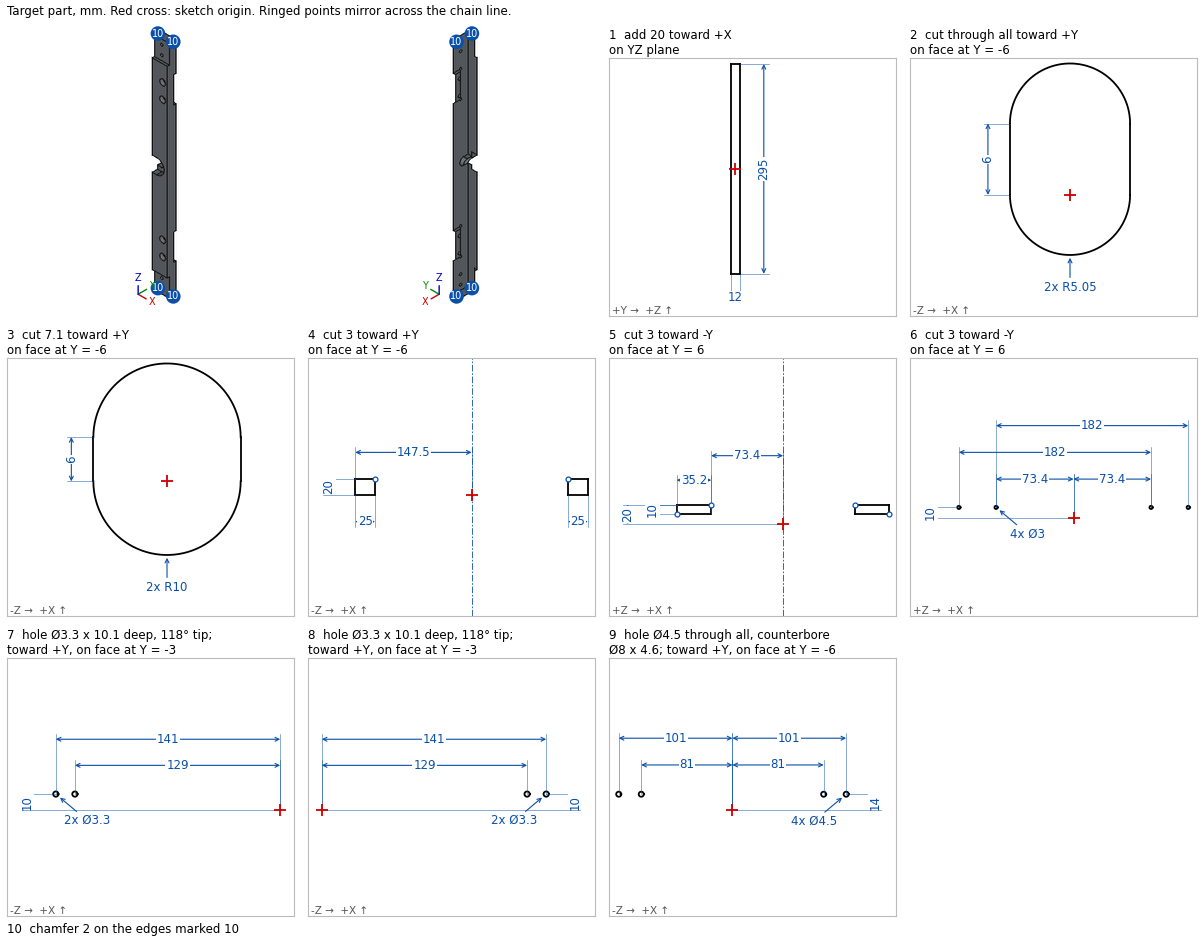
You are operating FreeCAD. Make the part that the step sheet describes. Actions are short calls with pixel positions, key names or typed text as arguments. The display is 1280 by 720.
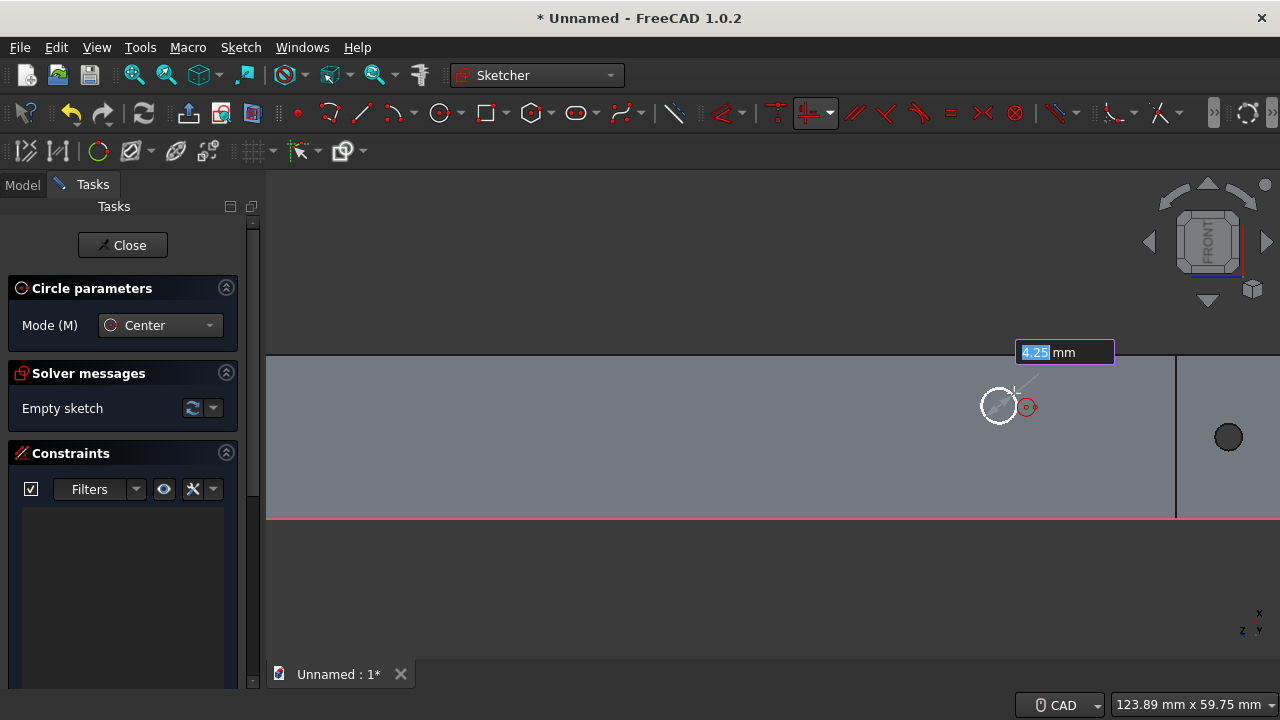
click(1013, 391)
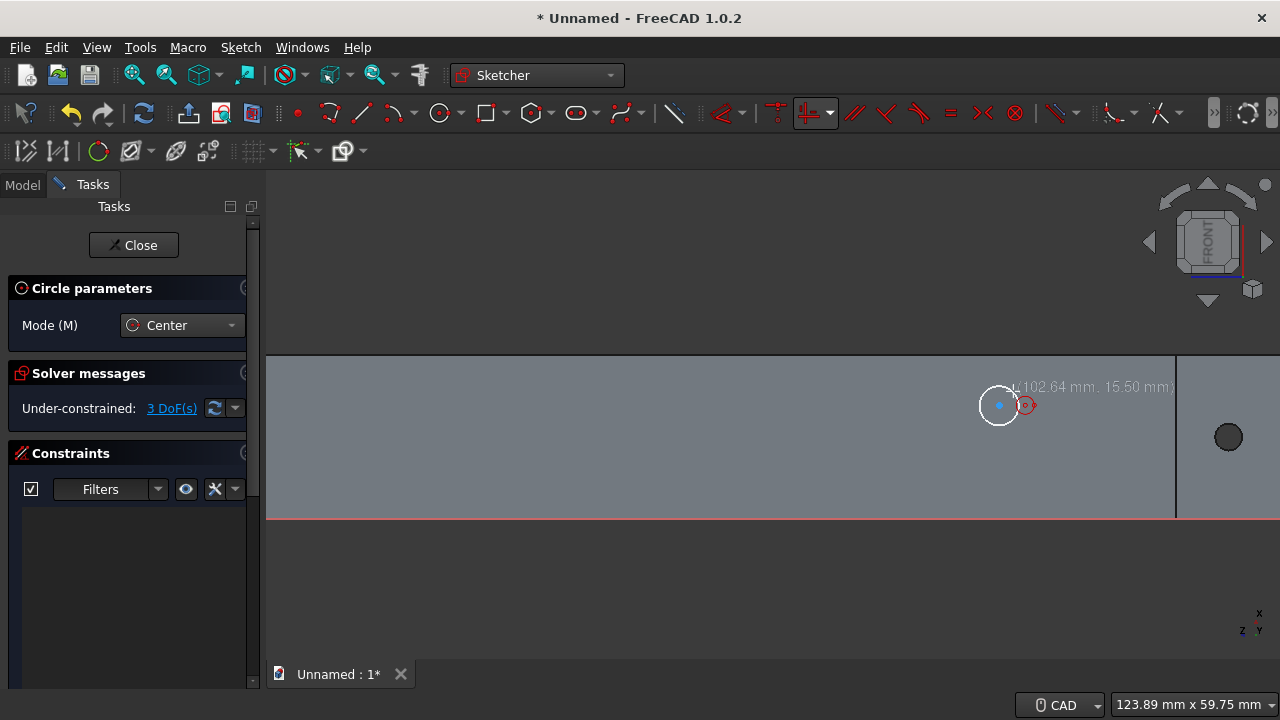
scroll(836, 404, up, 2)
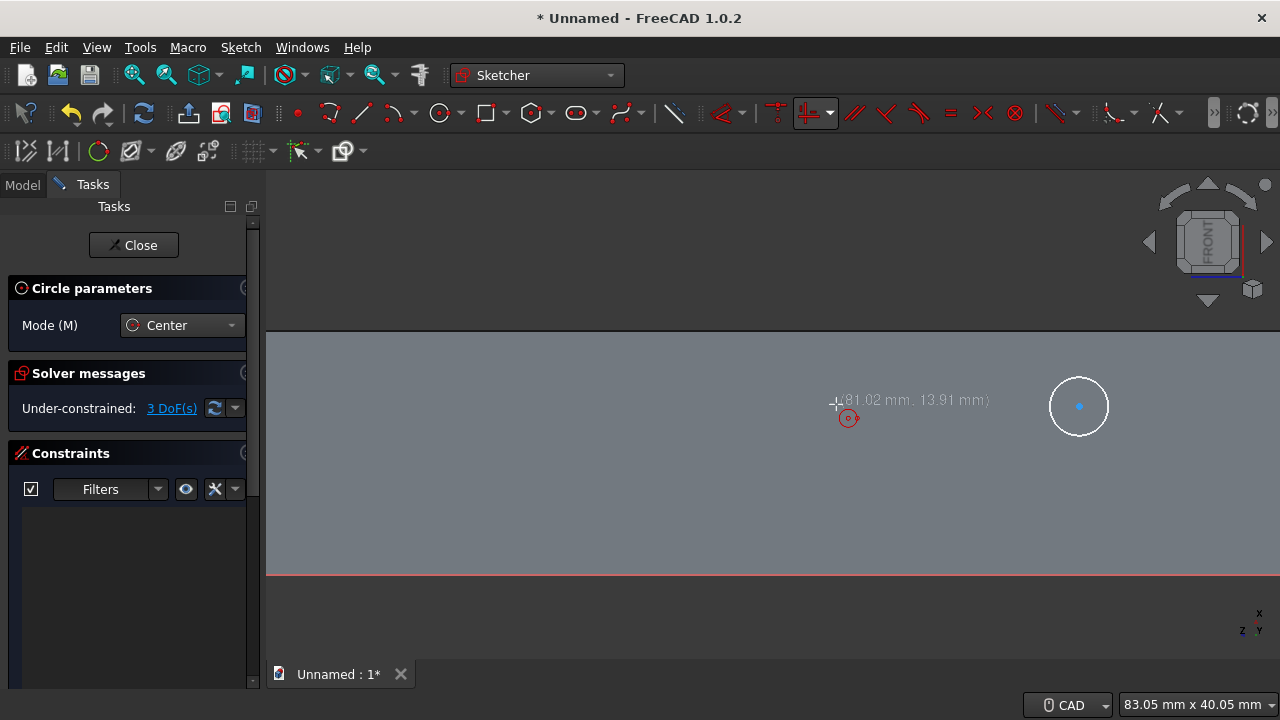
scroll(985, 394, down, 7)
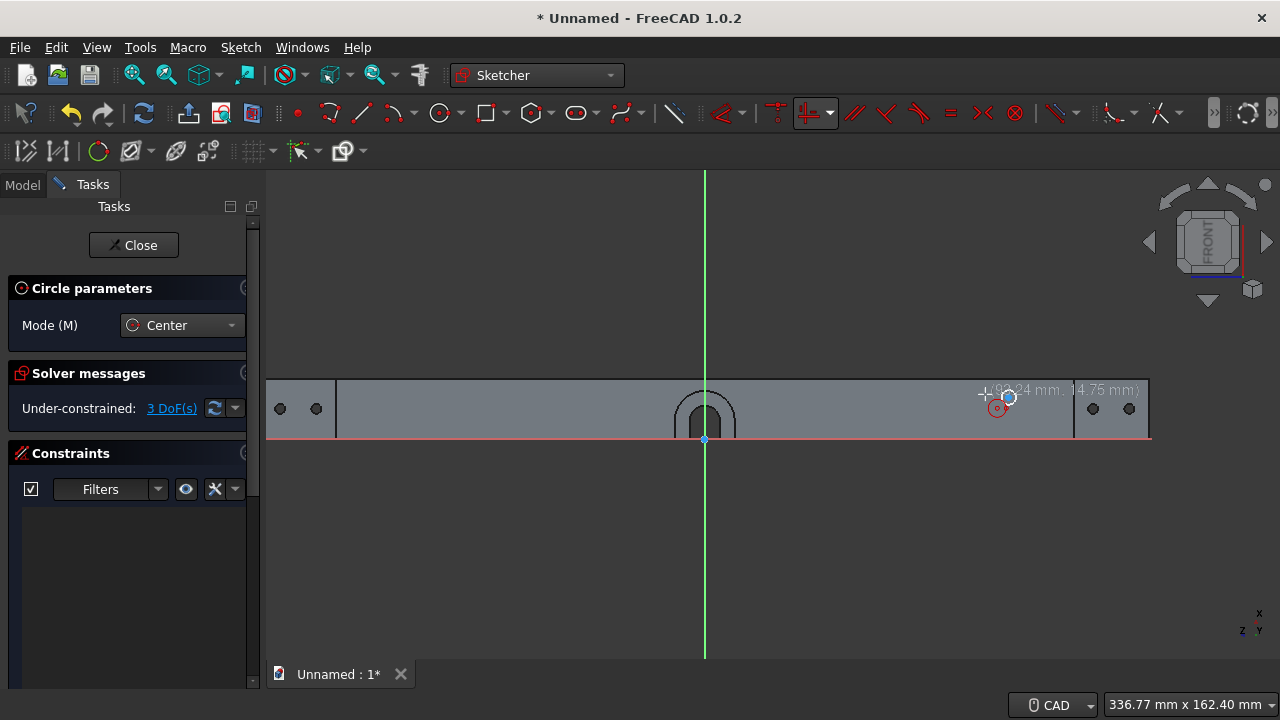
click(949, 397)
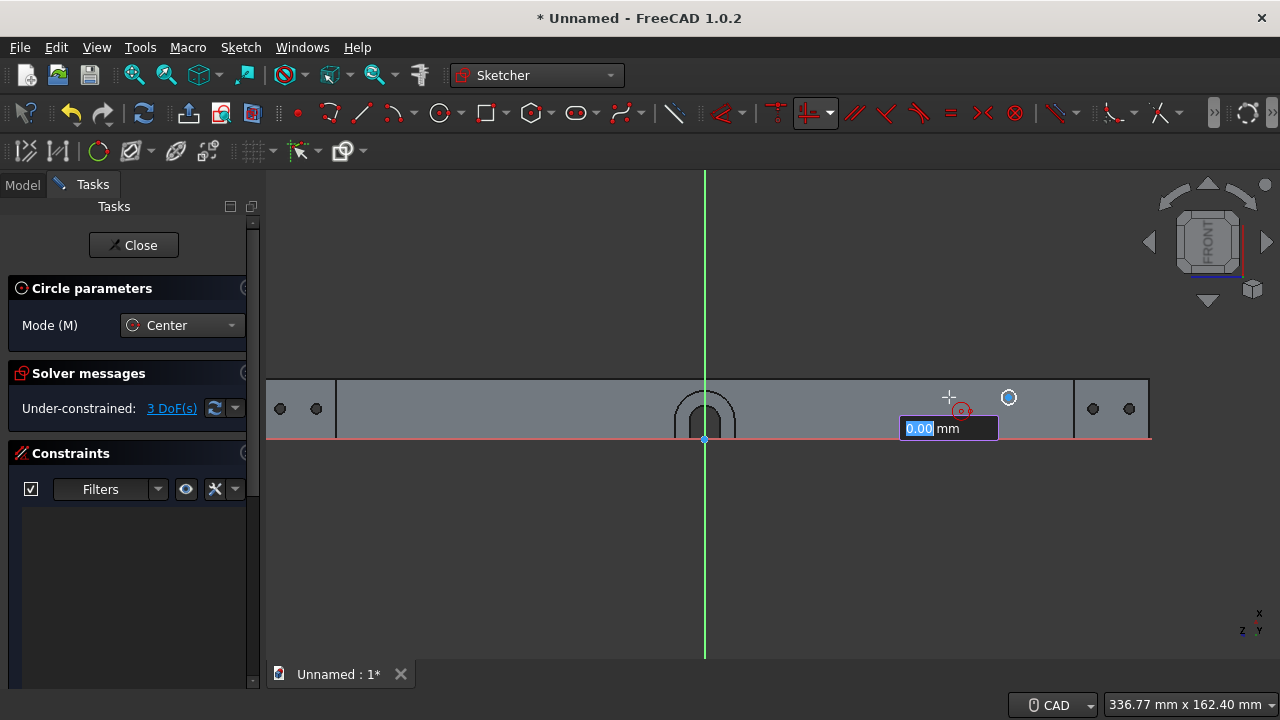
scroll(953, 392, up, 5)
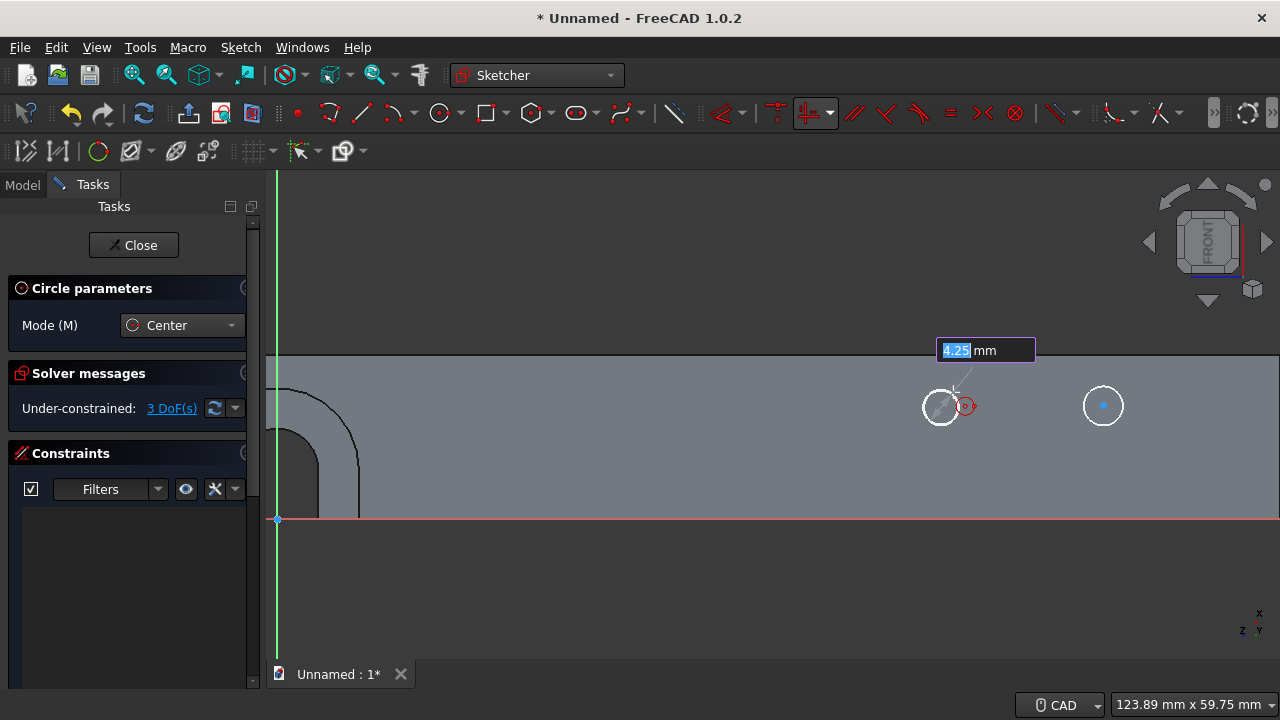
click(953, 391)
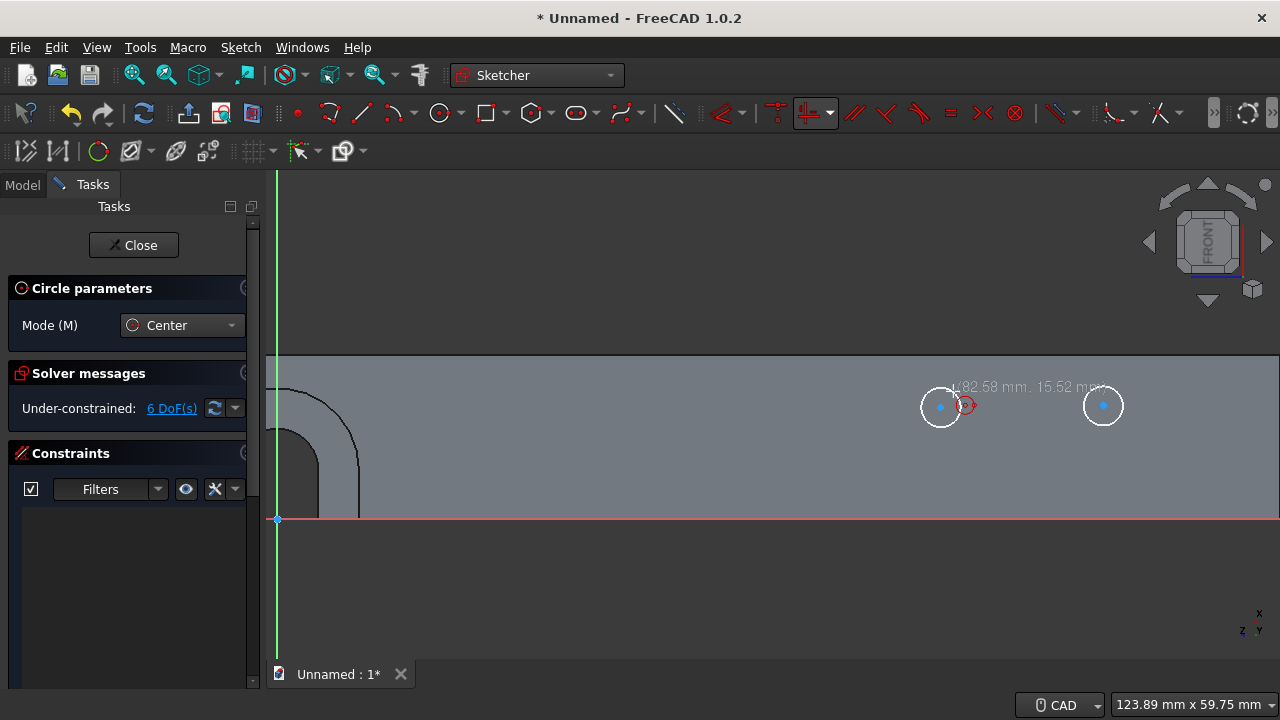
scroll(953, 392, down, 5)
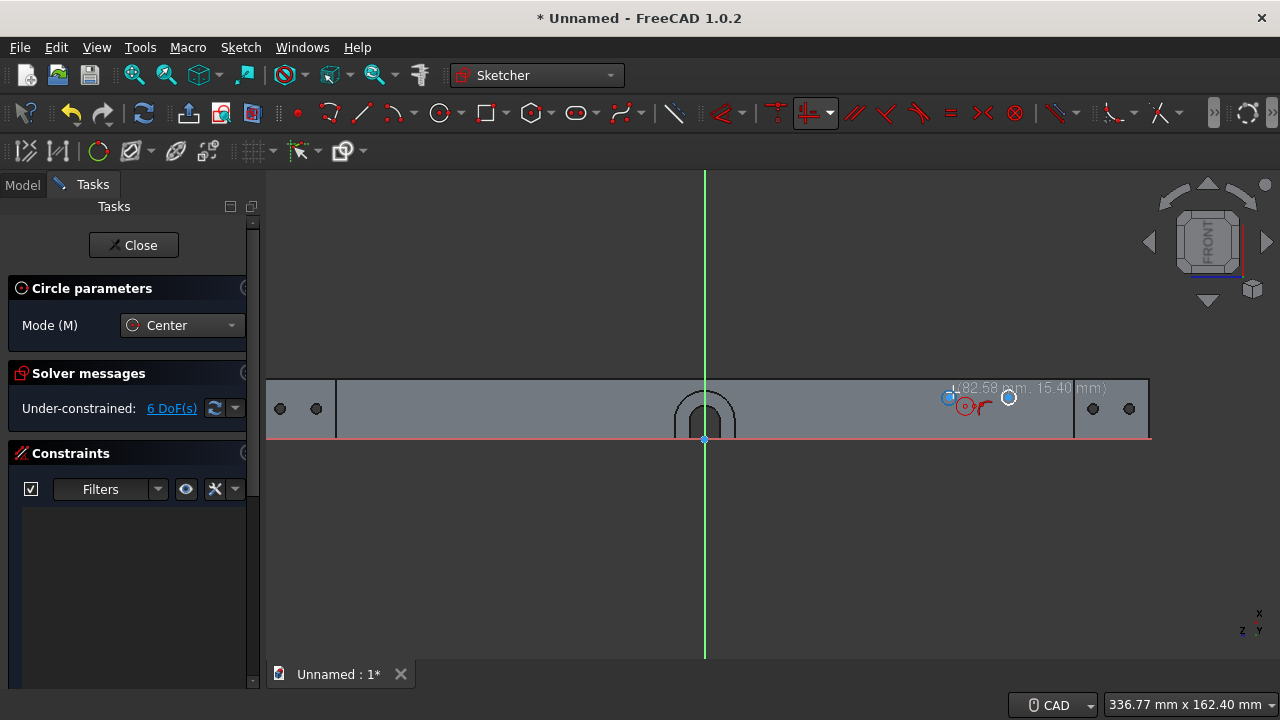
scroll(461, 397, up, 7)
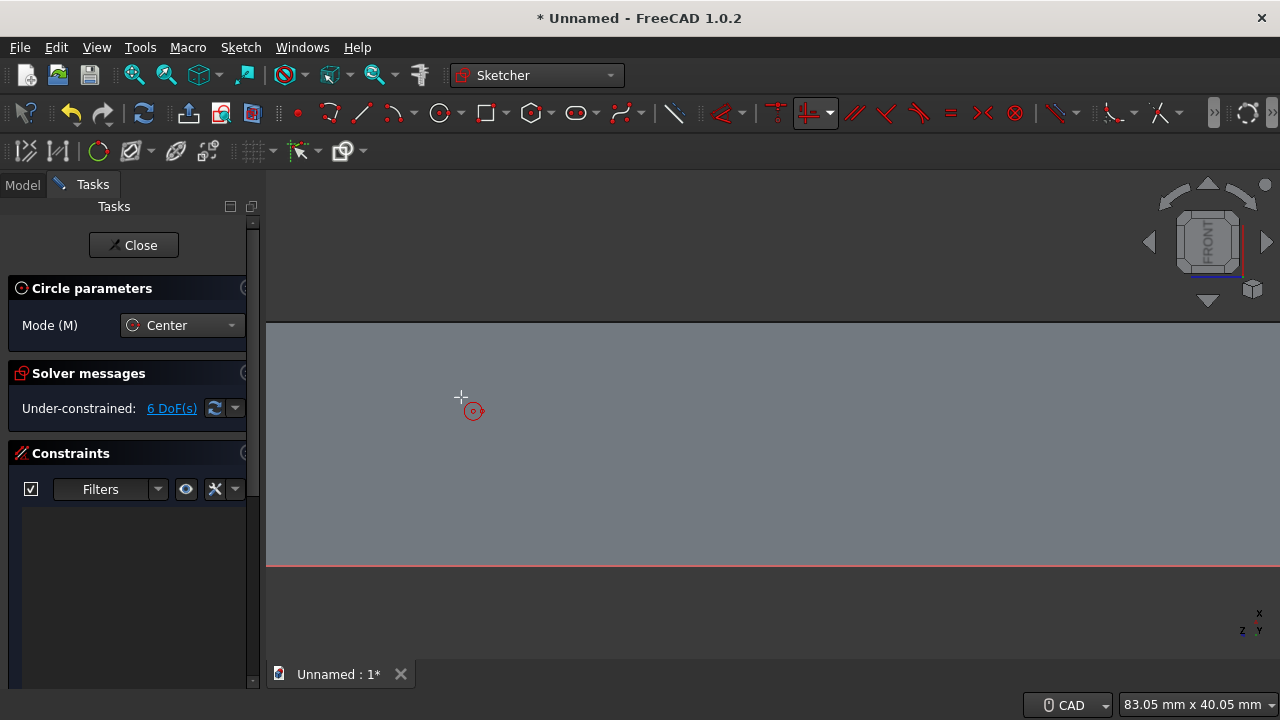
scroll(461, 397, down, 7)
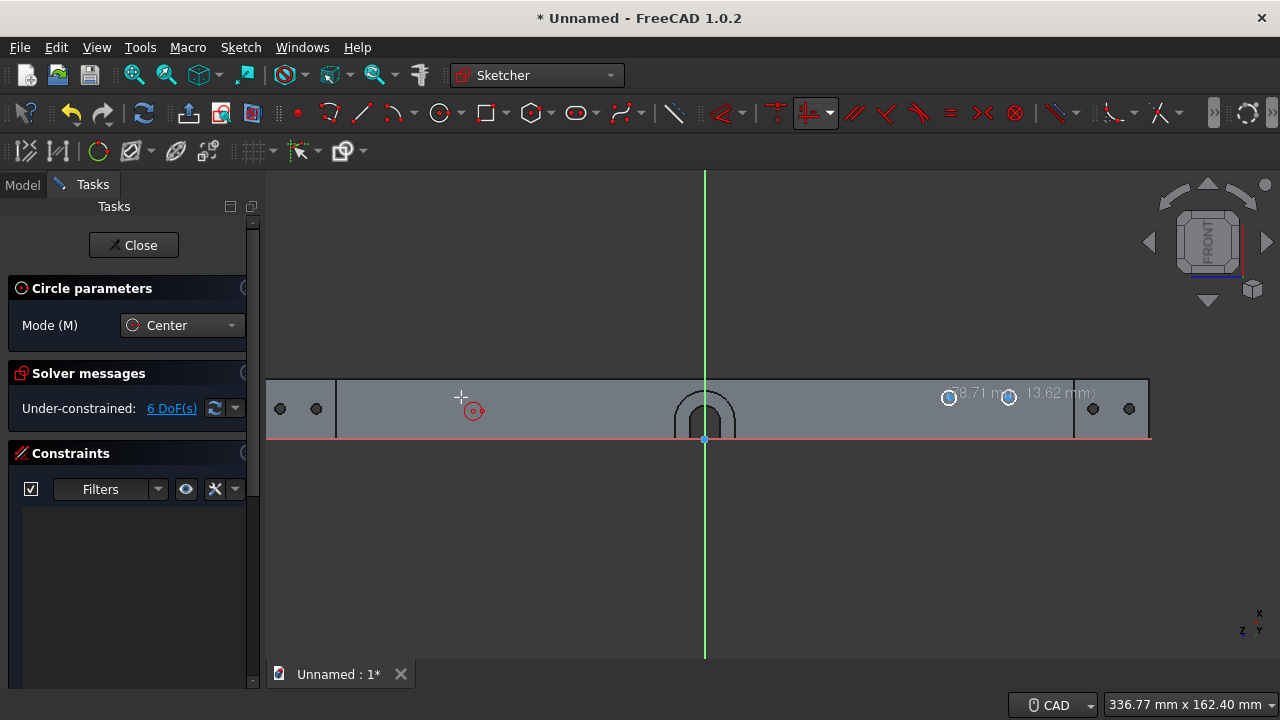
click(461, 397)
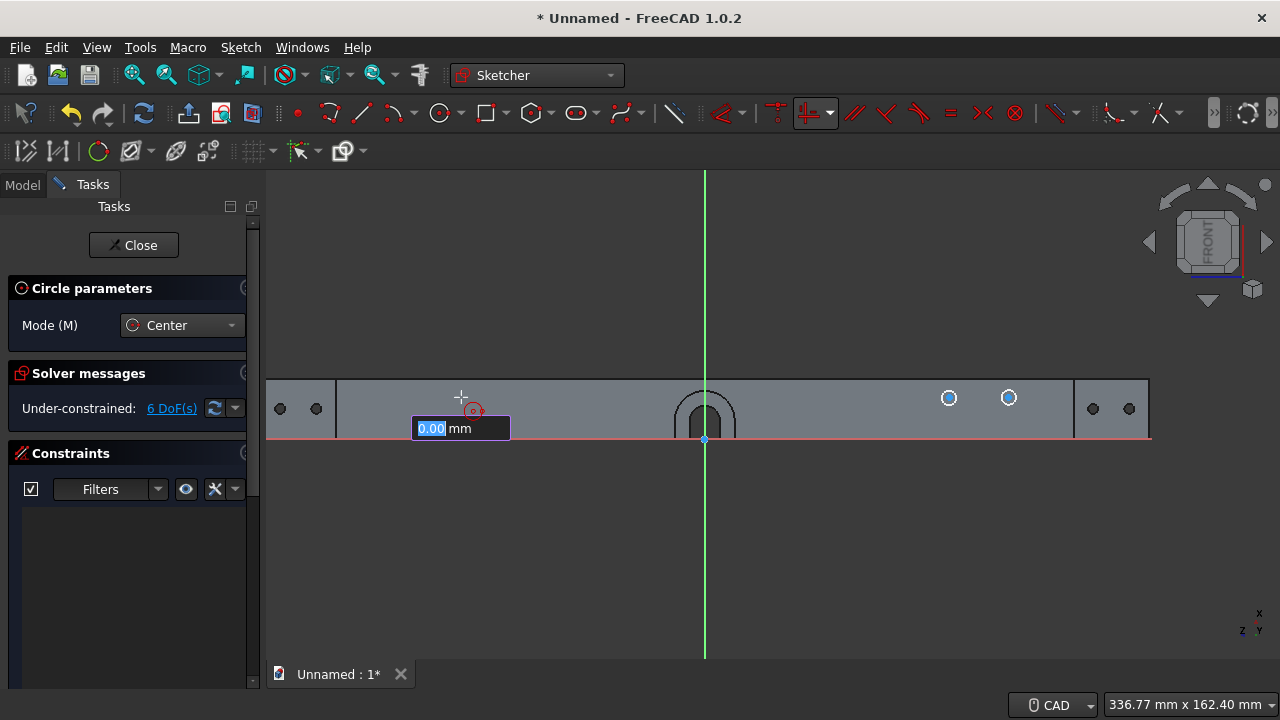
scroll(466, 392, up, 5)